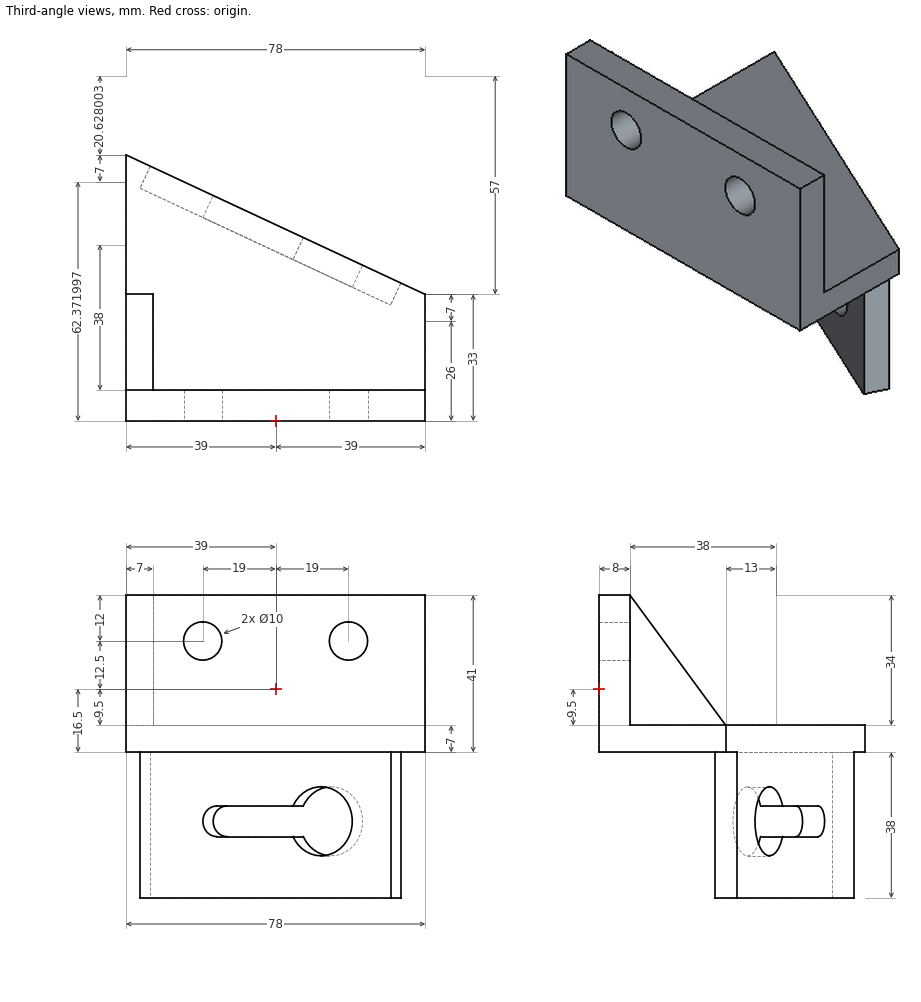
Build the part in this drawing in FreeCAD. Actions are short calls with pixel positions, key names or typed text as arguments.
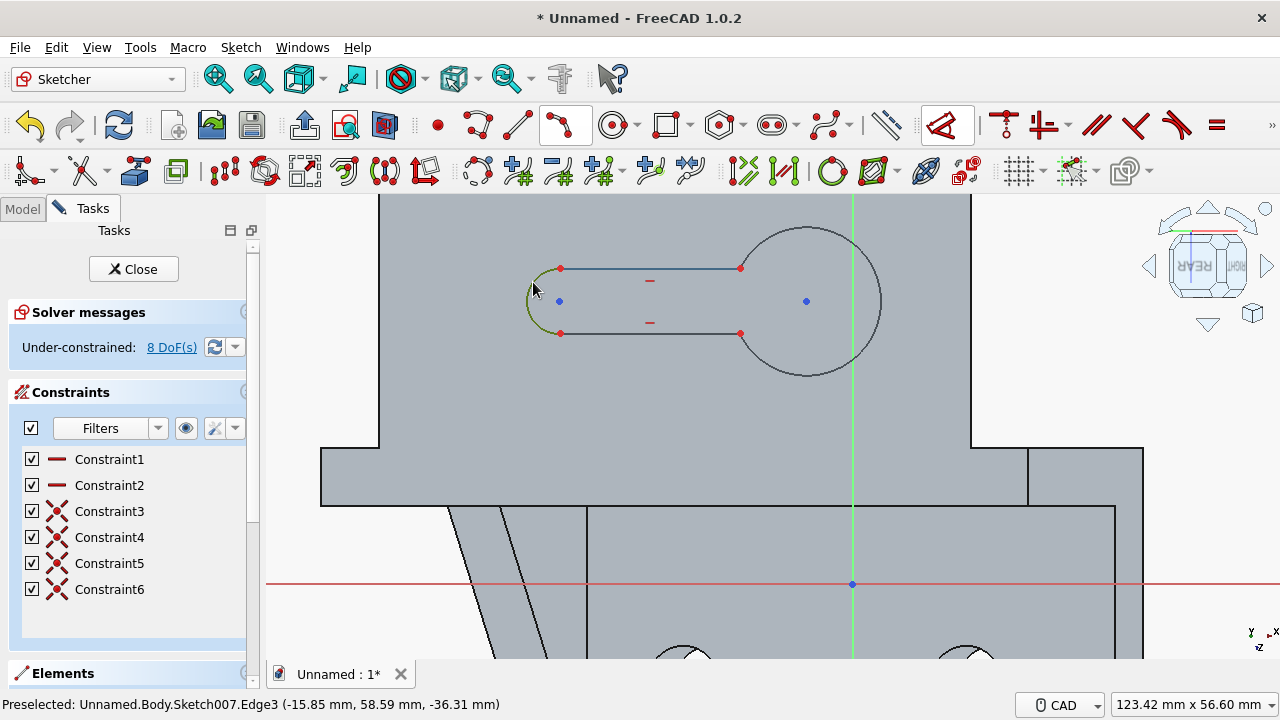
click(1178, 126)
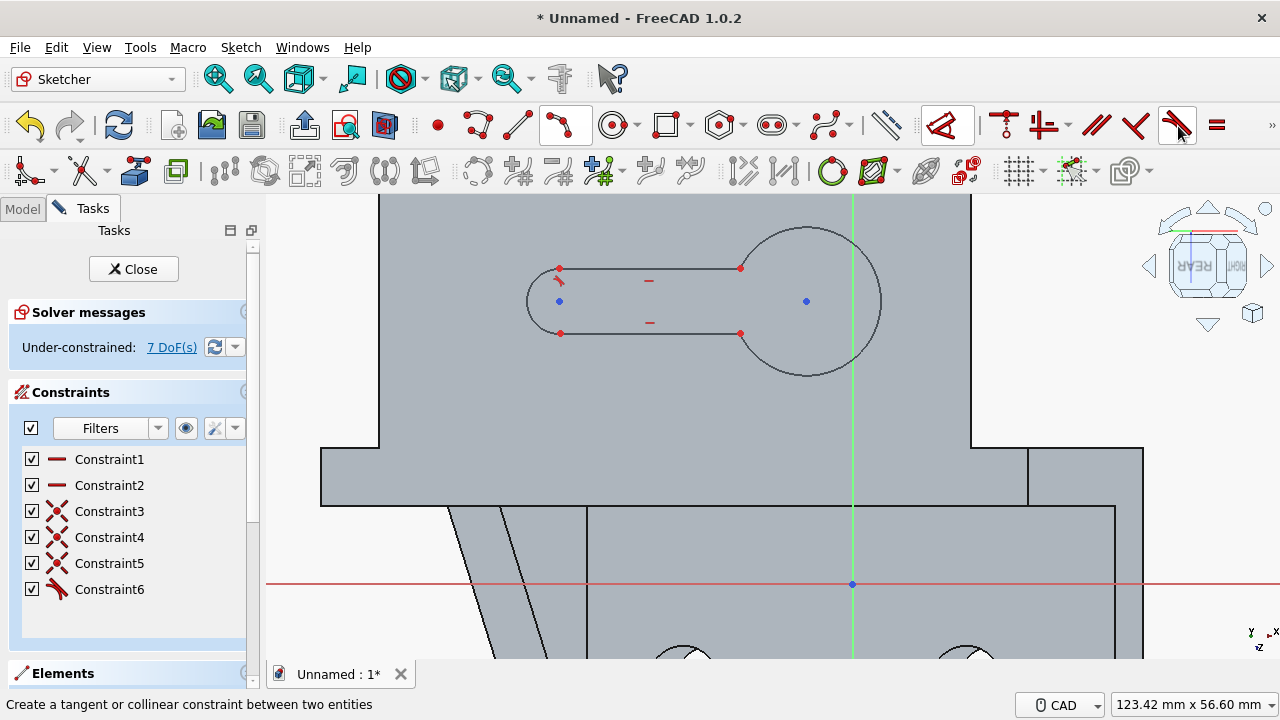
click(614, 334)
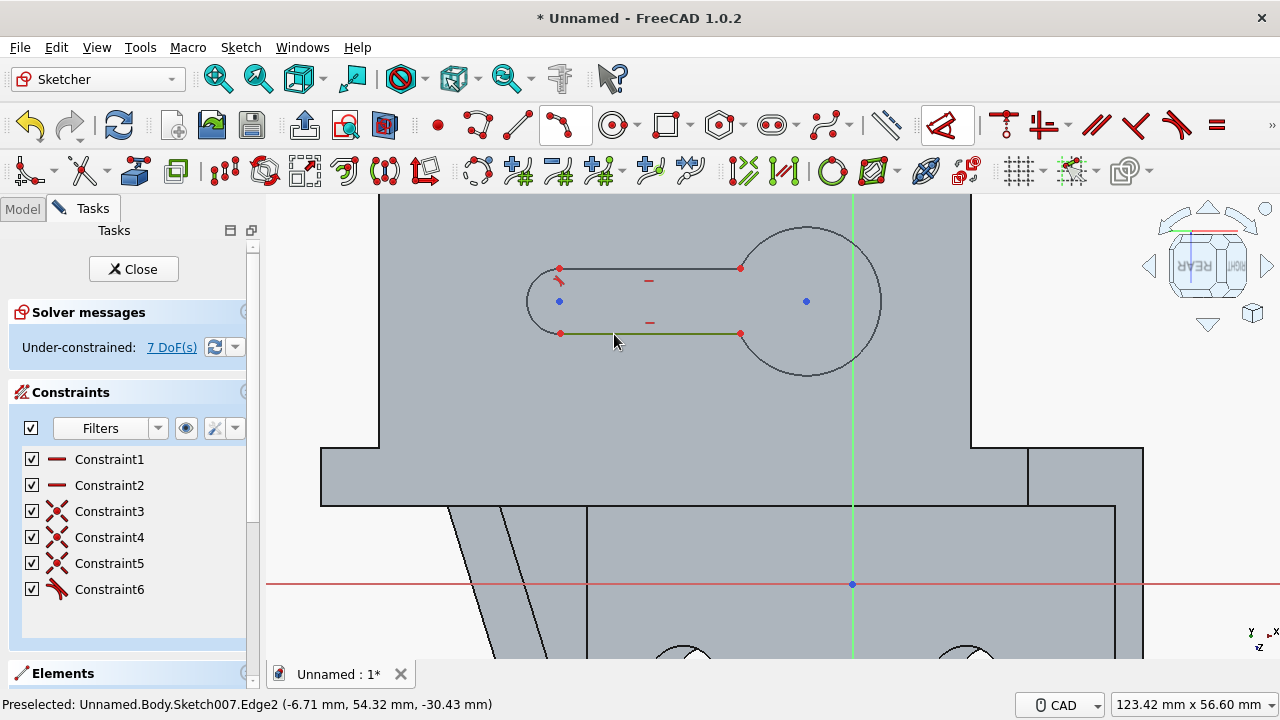
click(533, 283)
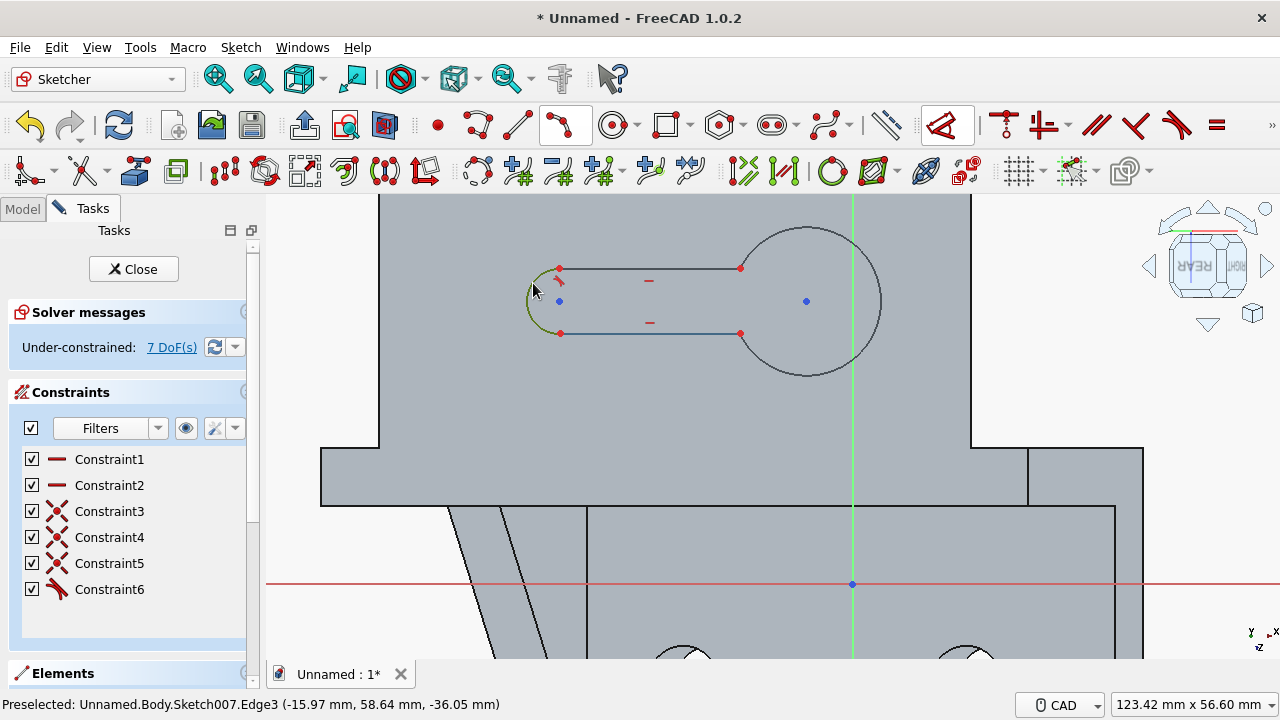
key(t)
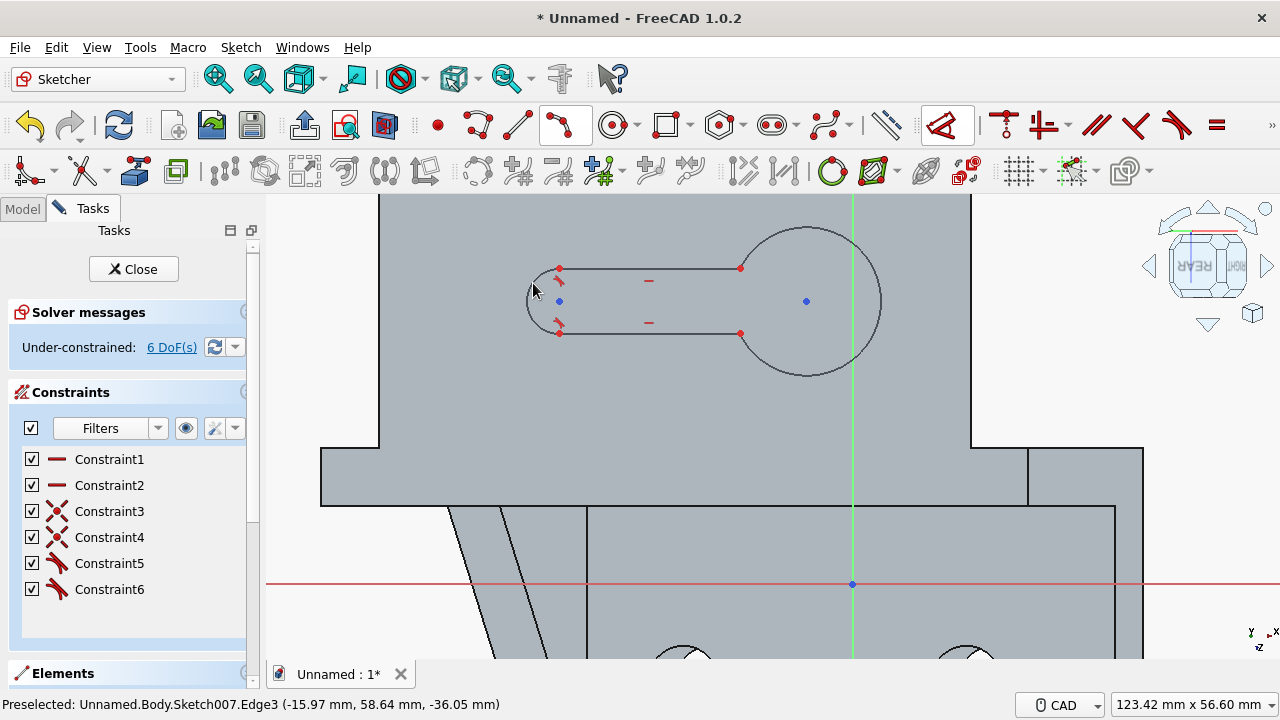
click(533, 282)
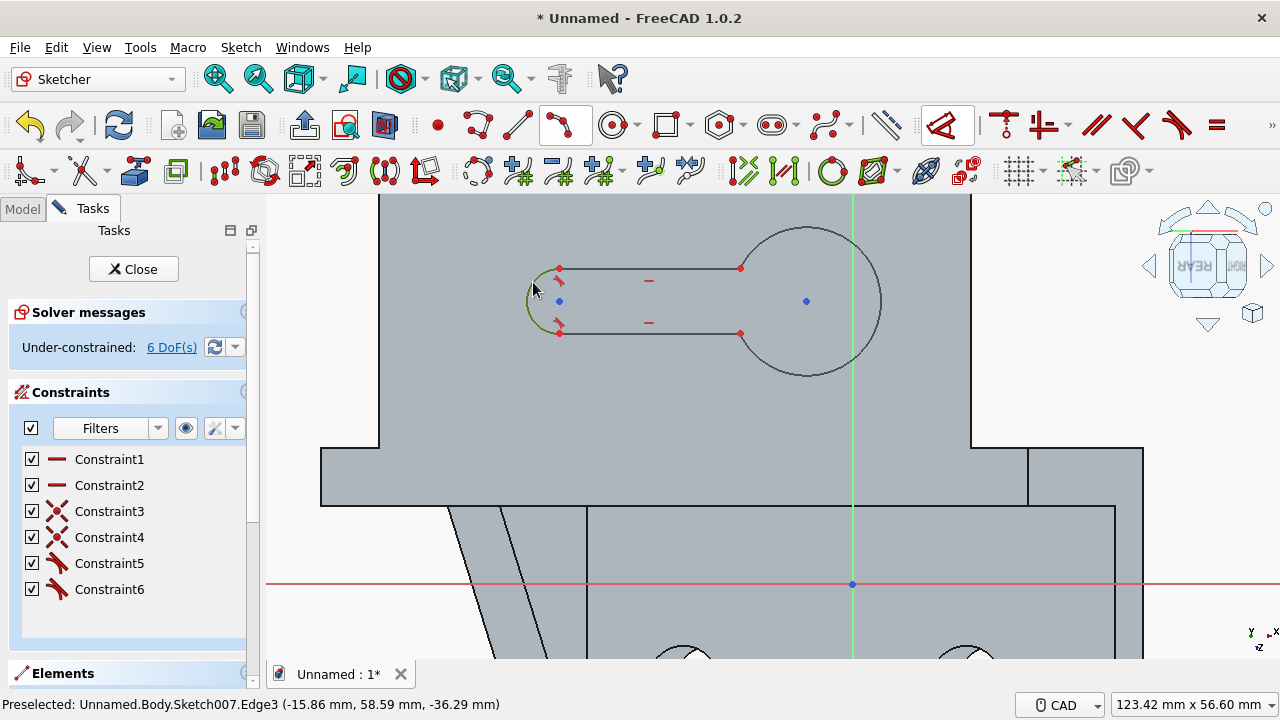
click(968, 126)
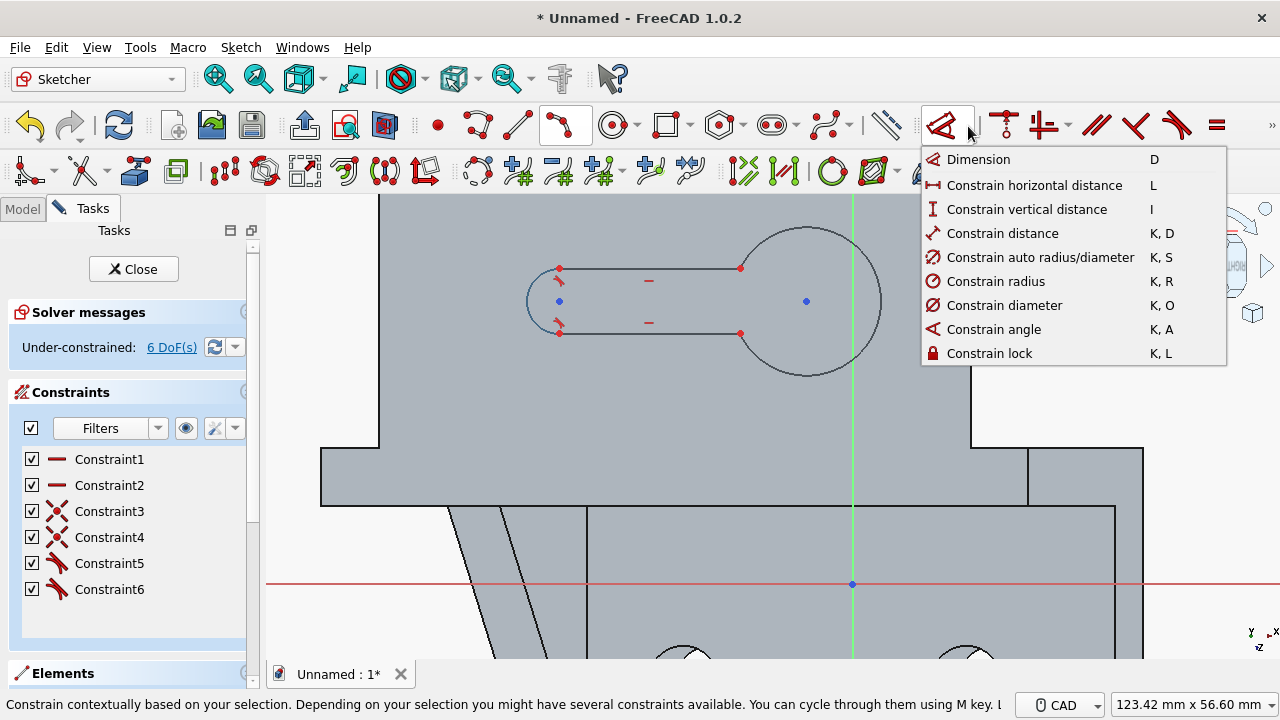
click(1074, 281)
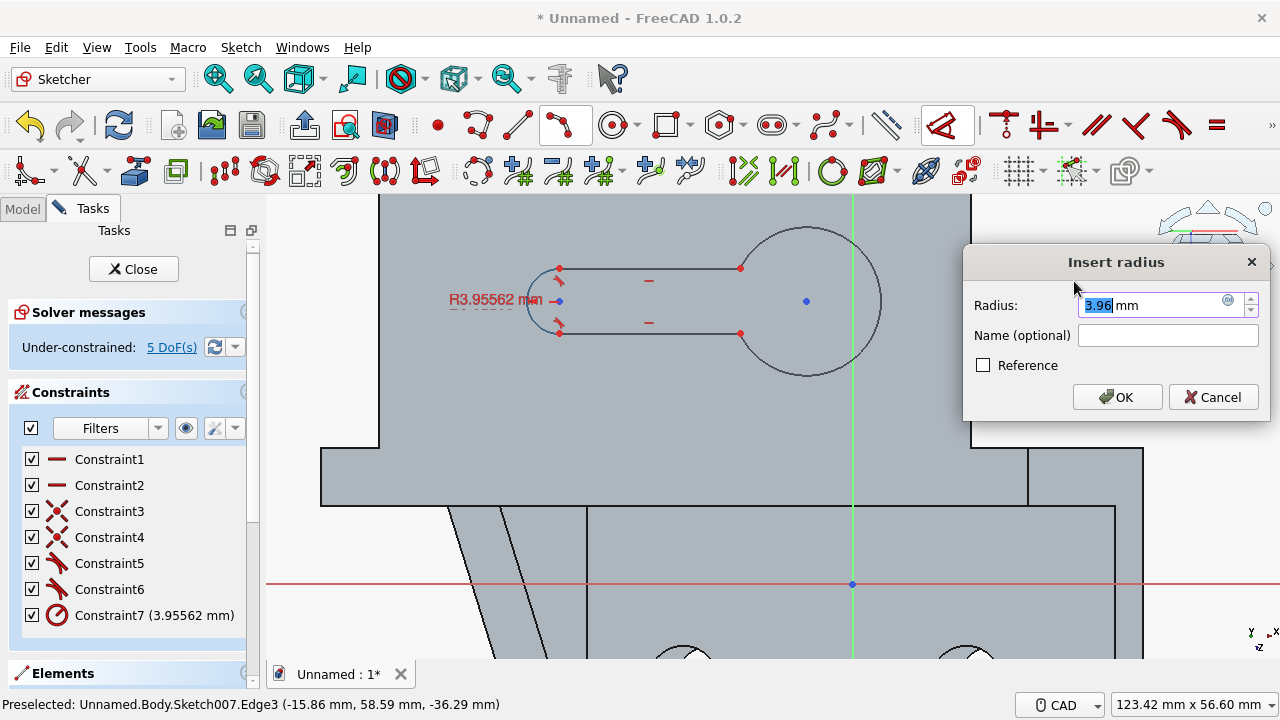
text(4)
key(Return)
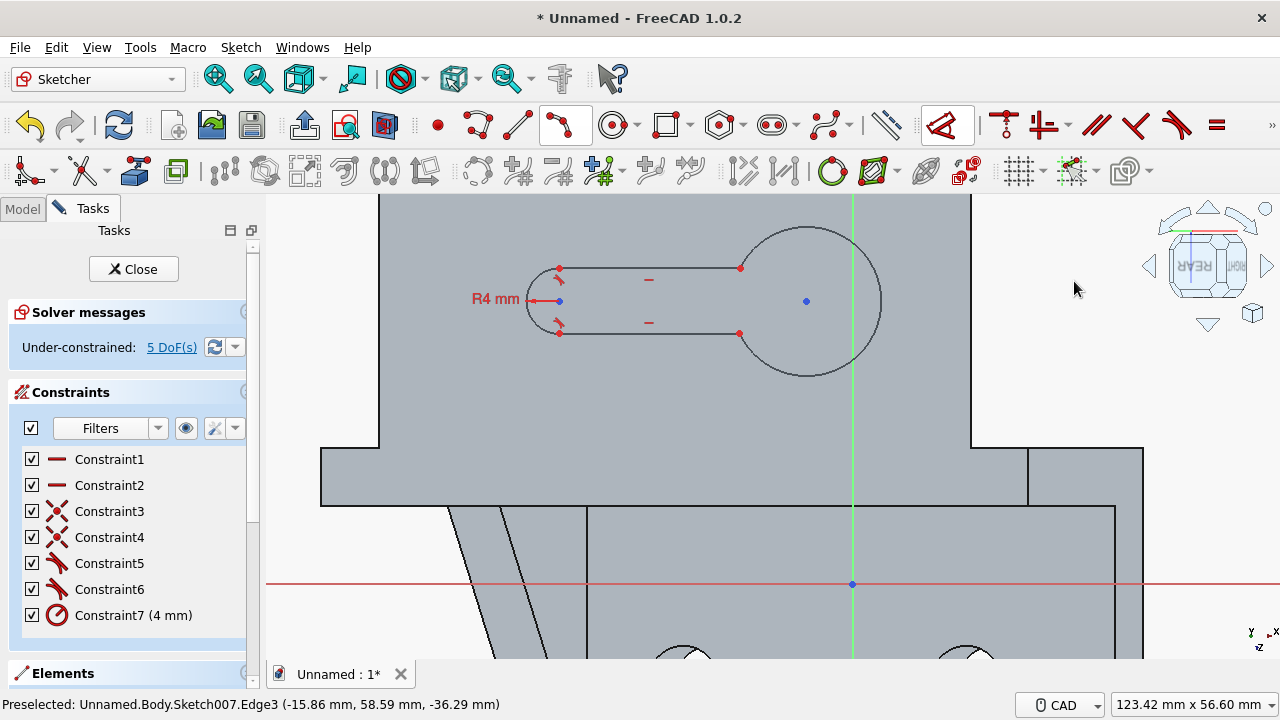
scroll(842, 367, up, 2)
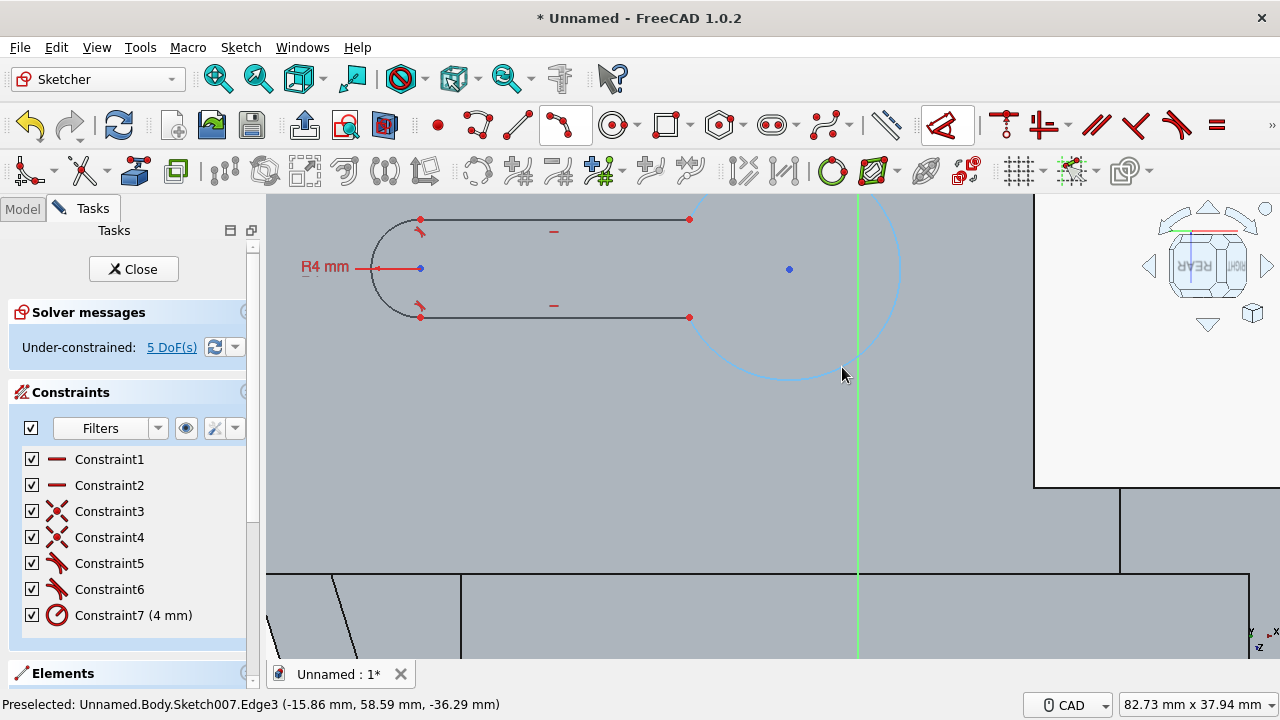
click(842, 367)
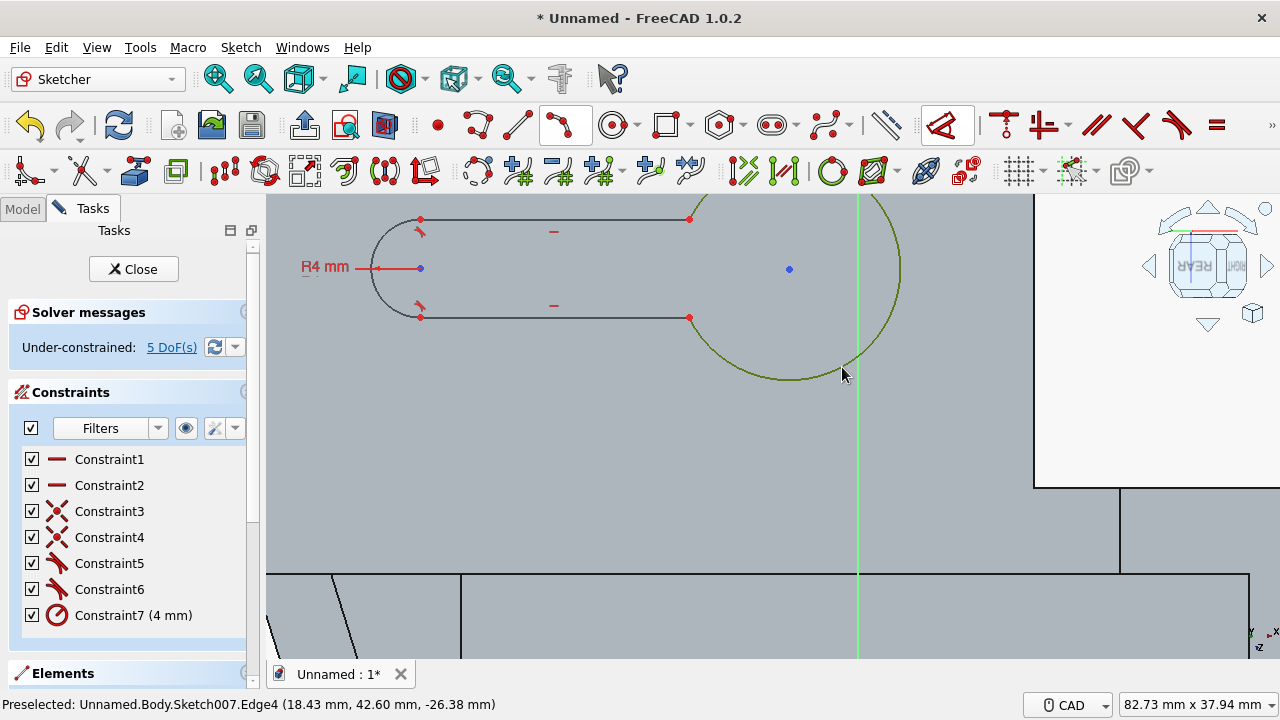
click(968, 126)